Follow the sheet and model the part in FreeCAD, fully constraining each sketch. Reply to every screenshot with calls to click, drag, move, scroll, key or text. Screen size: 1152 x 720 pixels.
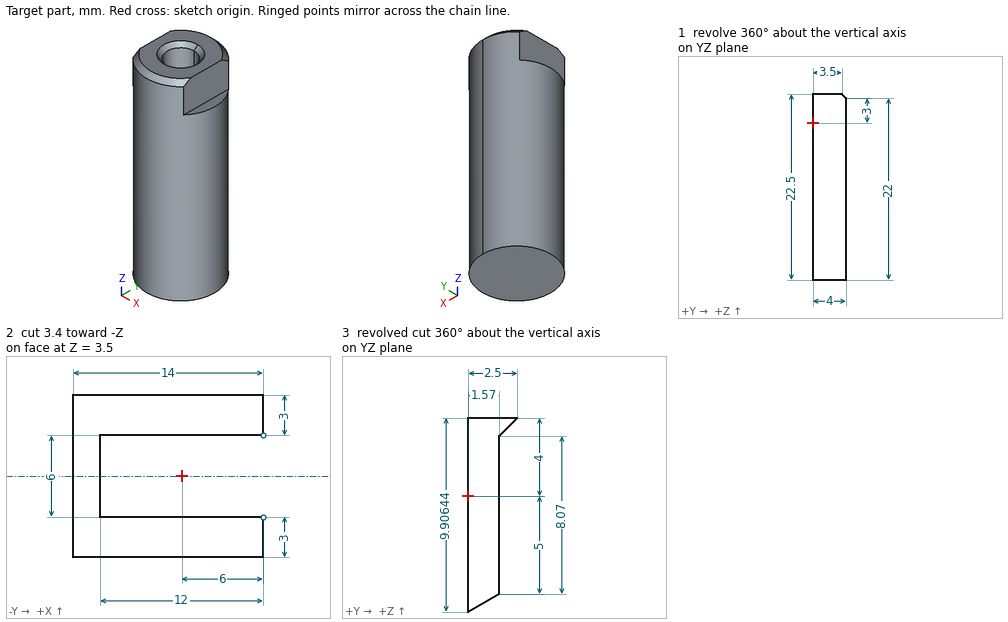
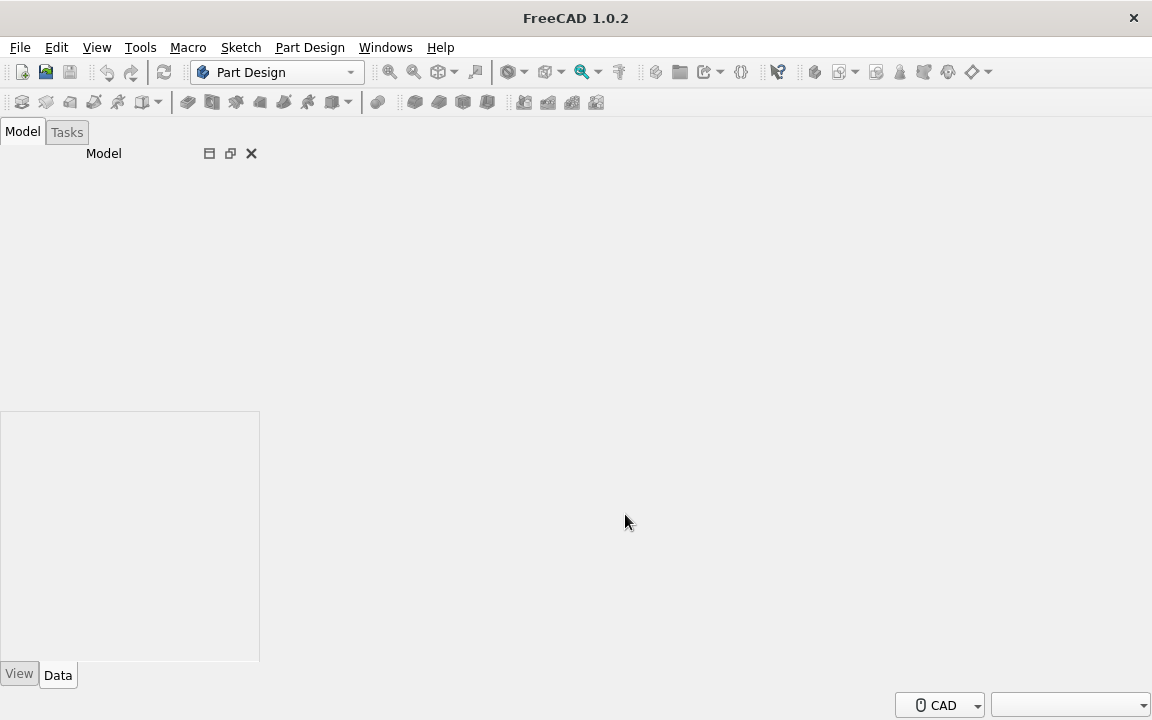
click(22, 72)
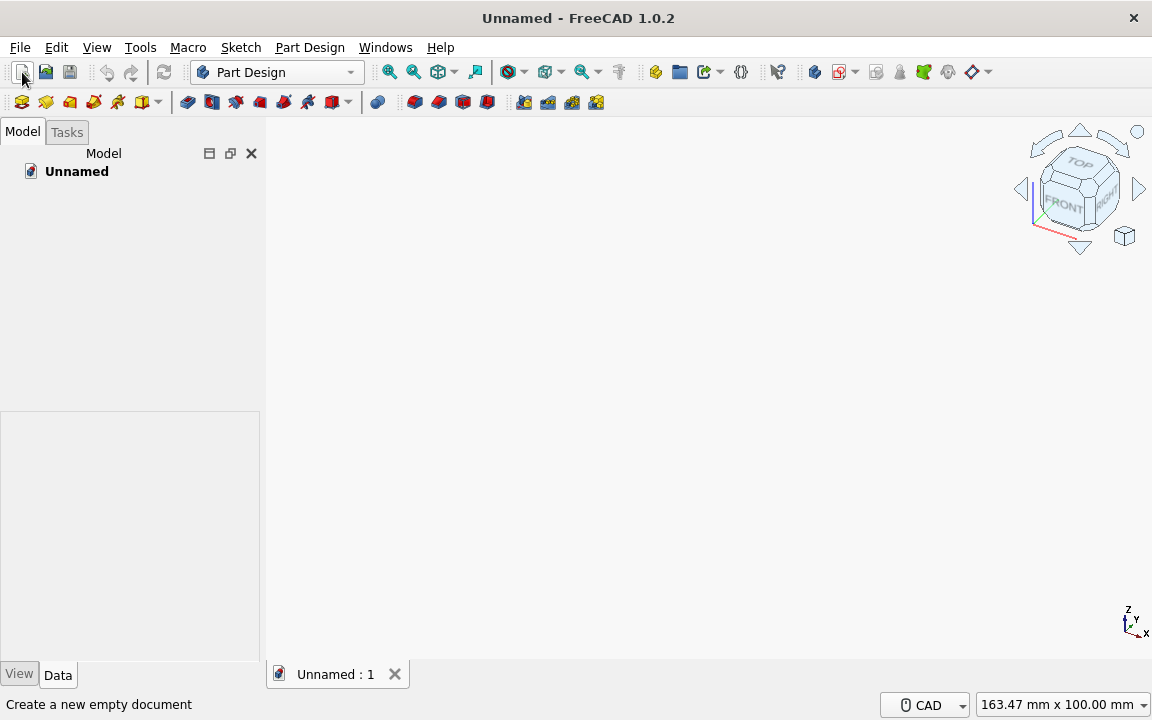
click(840, 72)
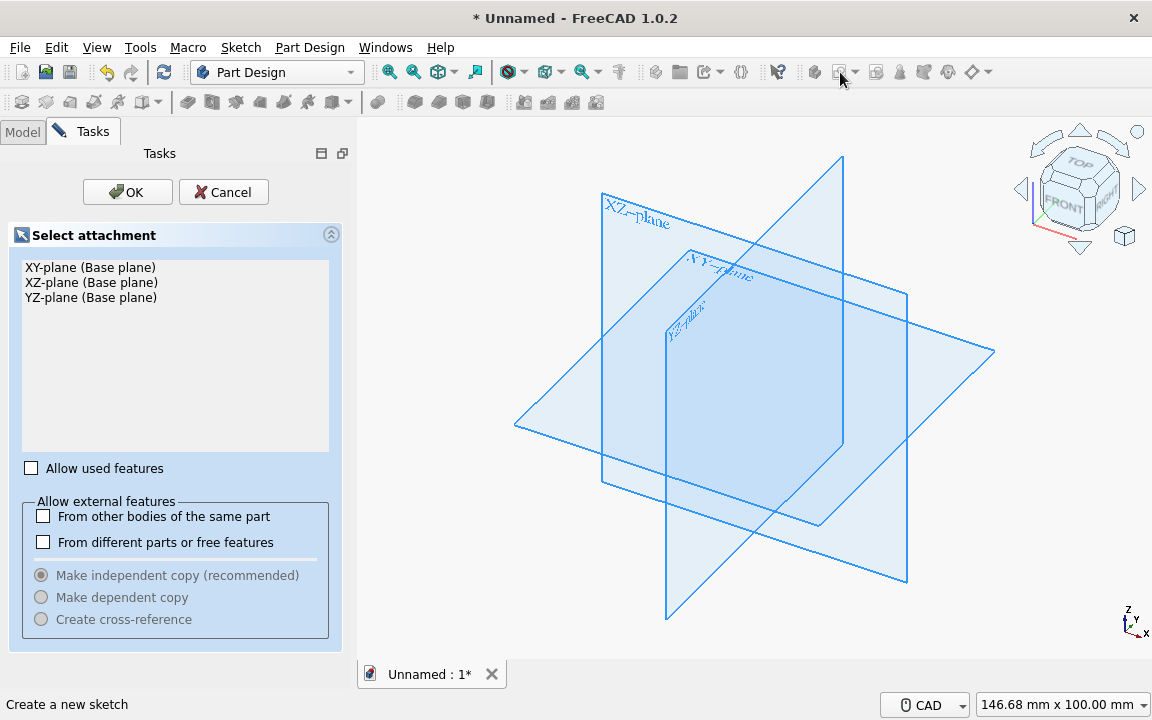
click(82, 298)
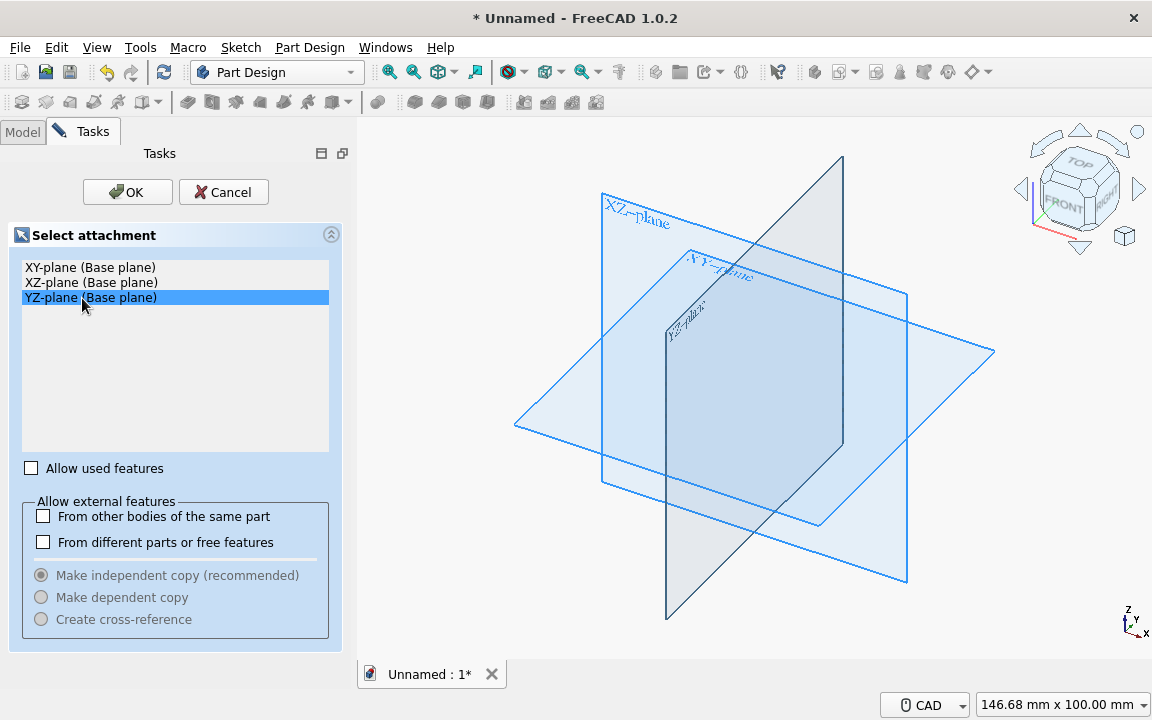
click(128, 192)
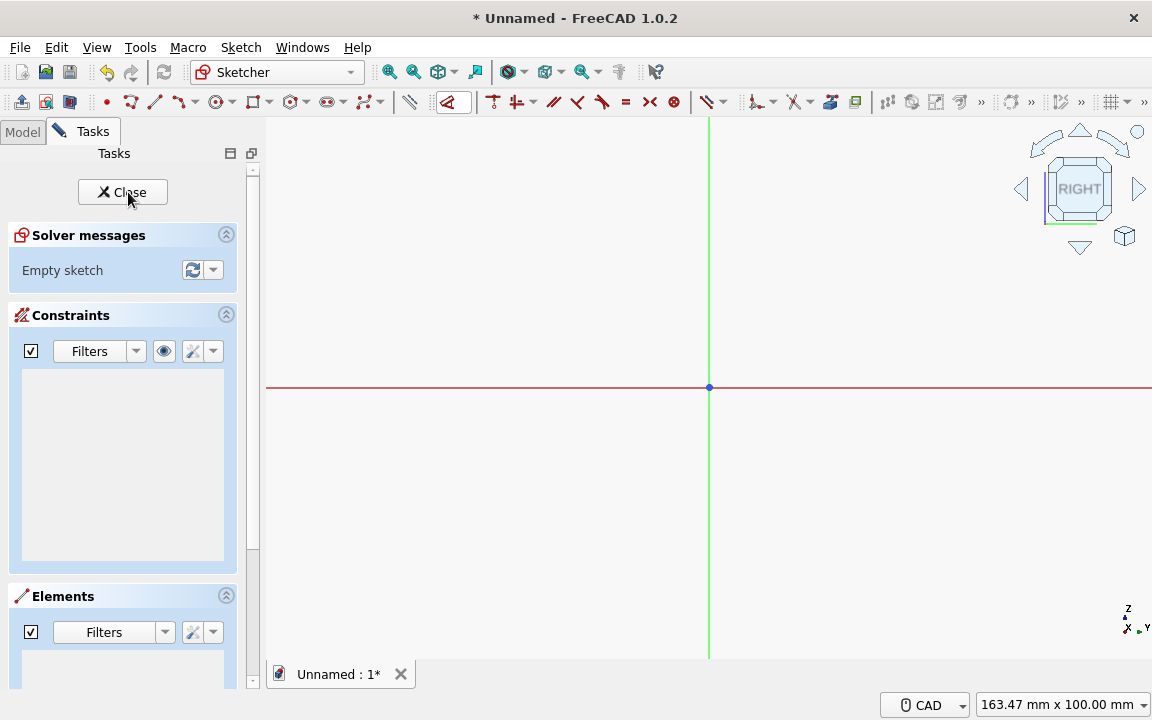
scroll(766, 454, up, 5)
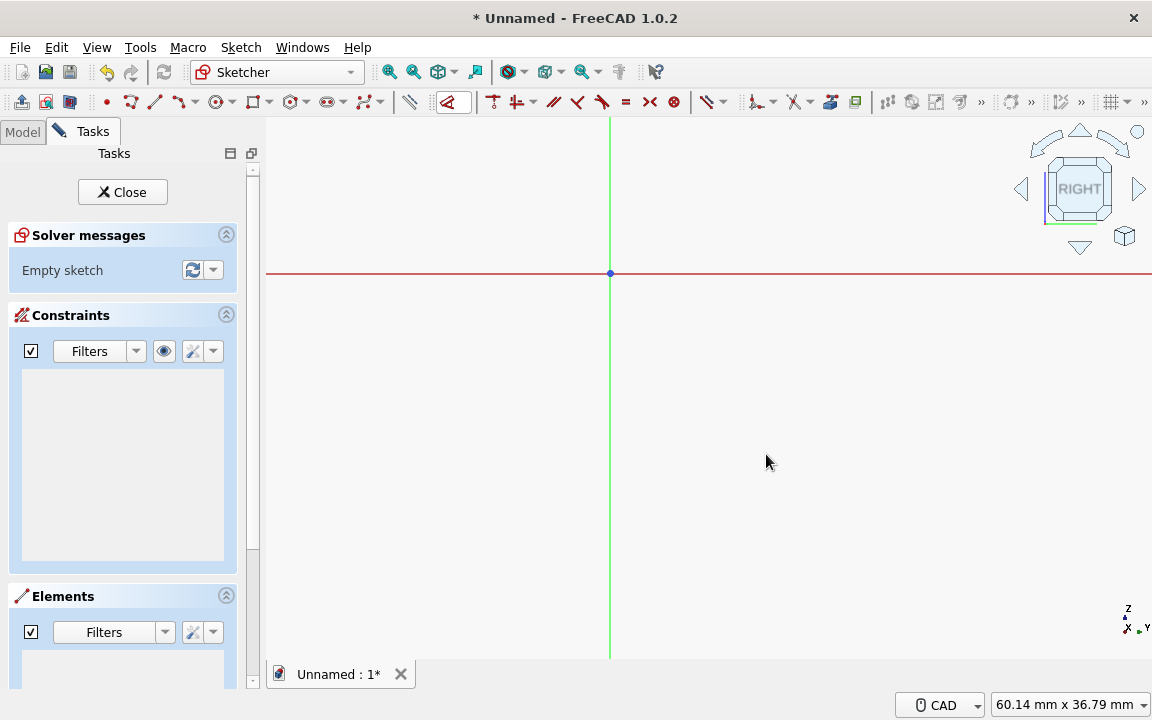
click(132, 102)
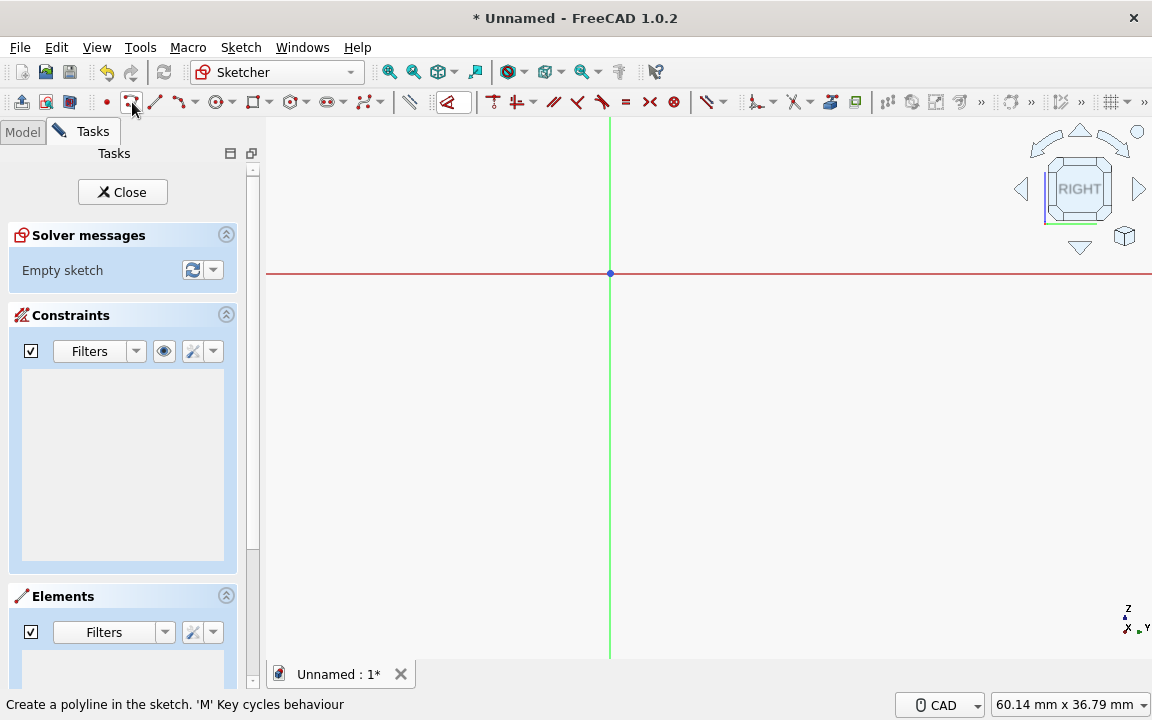
click(610, 222)
click(619, 553)
click(669, 553)
click(669, 229)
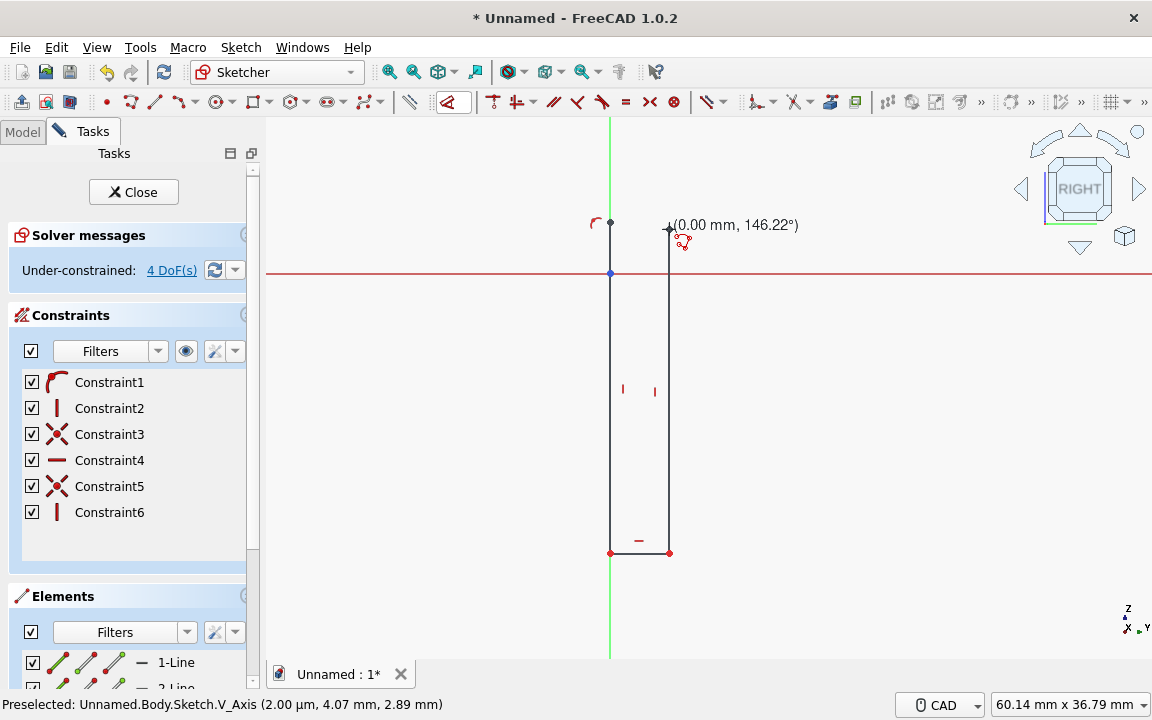
scroll(662, 222, up, 3)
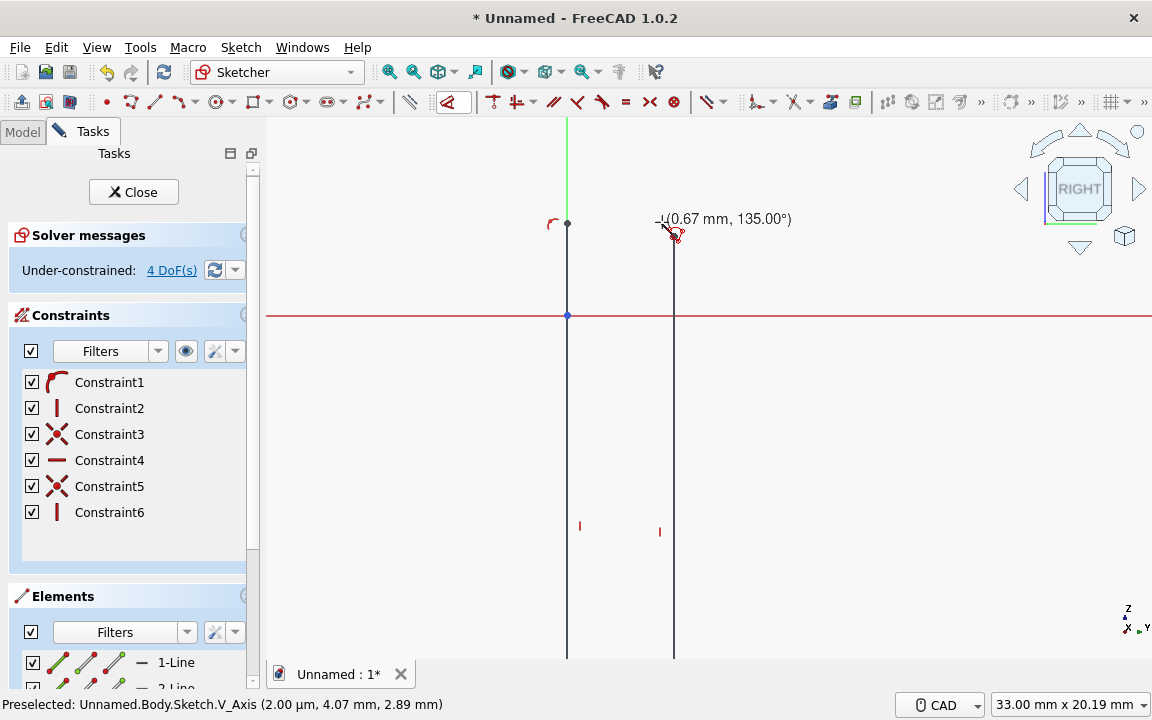
click(661, 222)
click(567, 224)
key(Escape)
key(Escape)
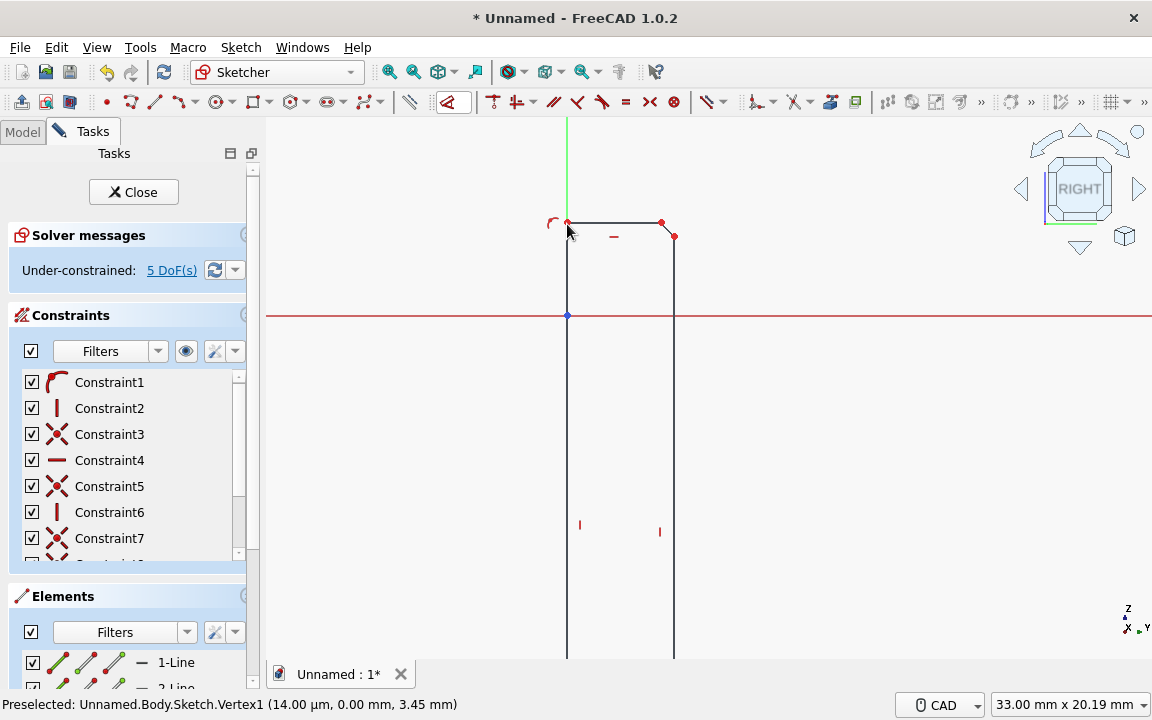
click(448, 102)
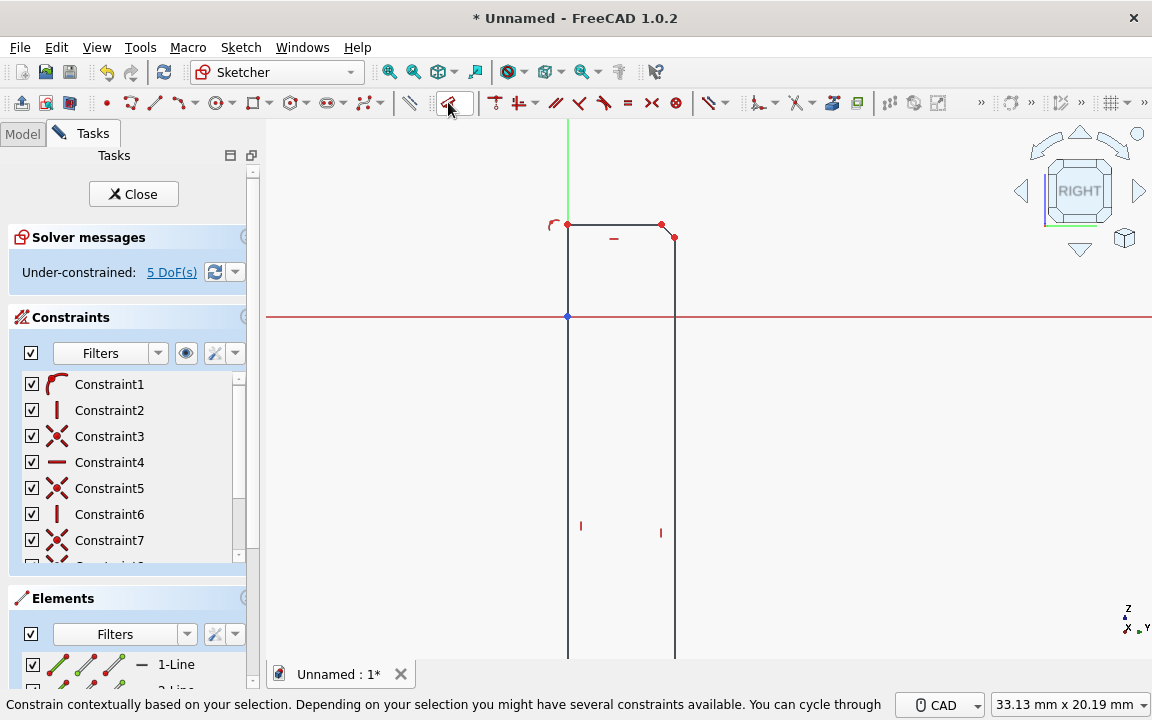
scroll(664, 224, down, 3)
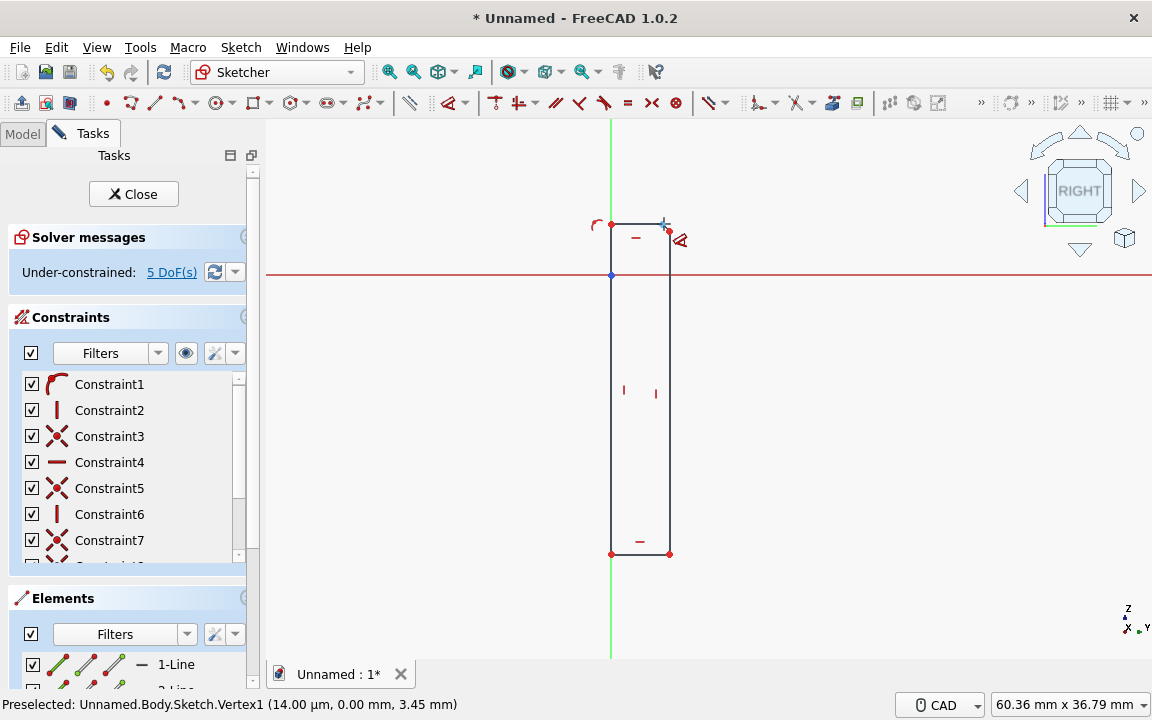
click(629, 555)
click(641, 589)